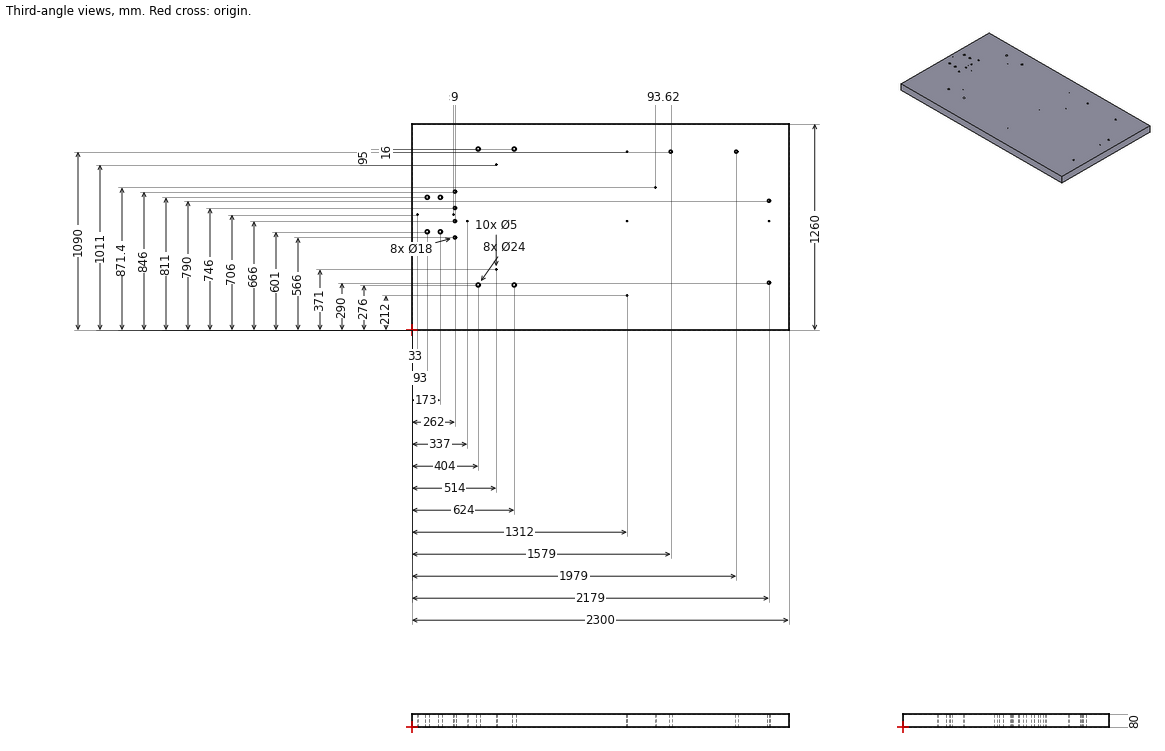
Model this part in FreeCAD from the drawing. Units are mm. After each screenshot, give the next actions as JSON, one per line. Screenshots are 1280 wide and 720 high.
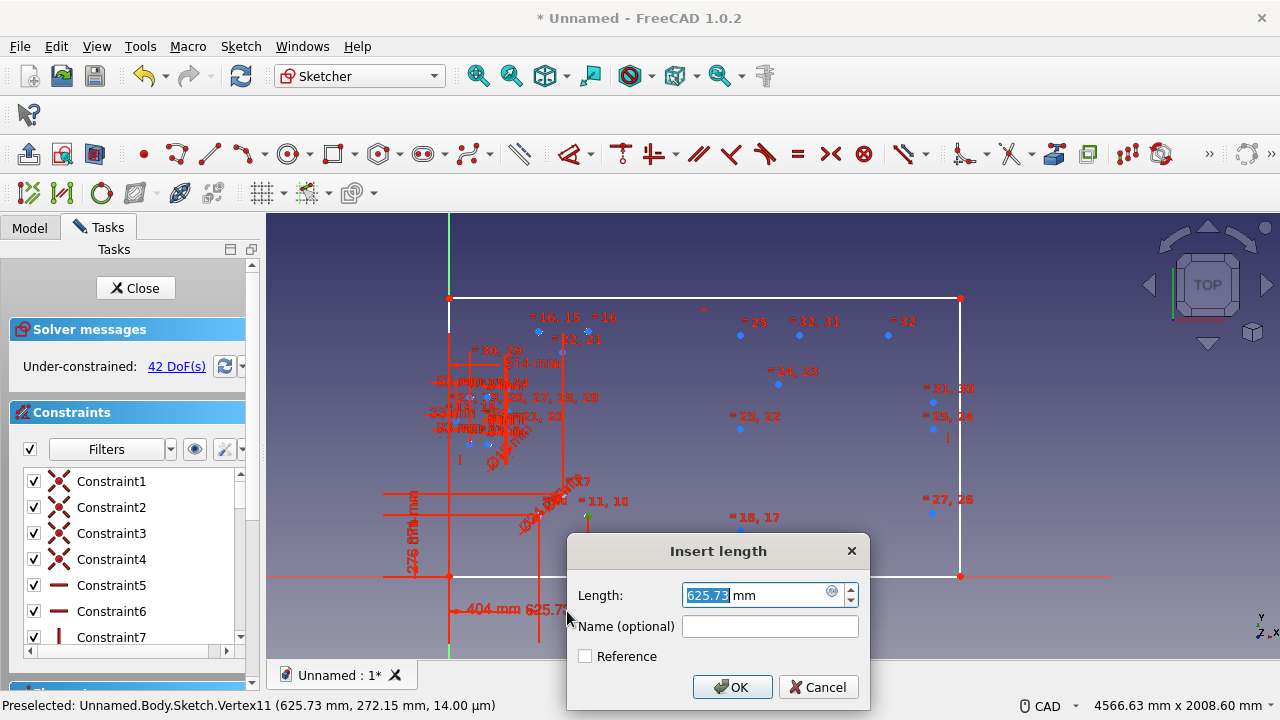
{"action": "type", "text": "624"}
{"action": "key", "text": "Return"}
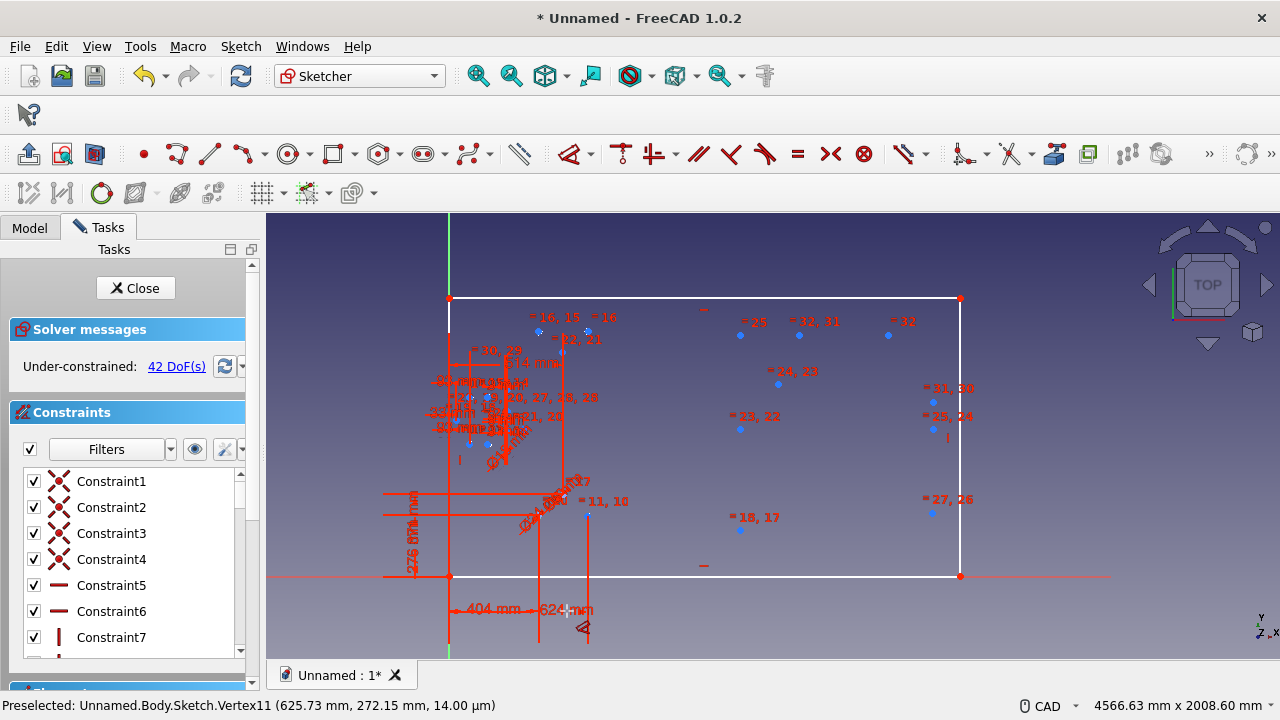
{"action": "left_click", "coordinate": [588, 516]}
{"action": "left_click", "coordinate": [622, 546]}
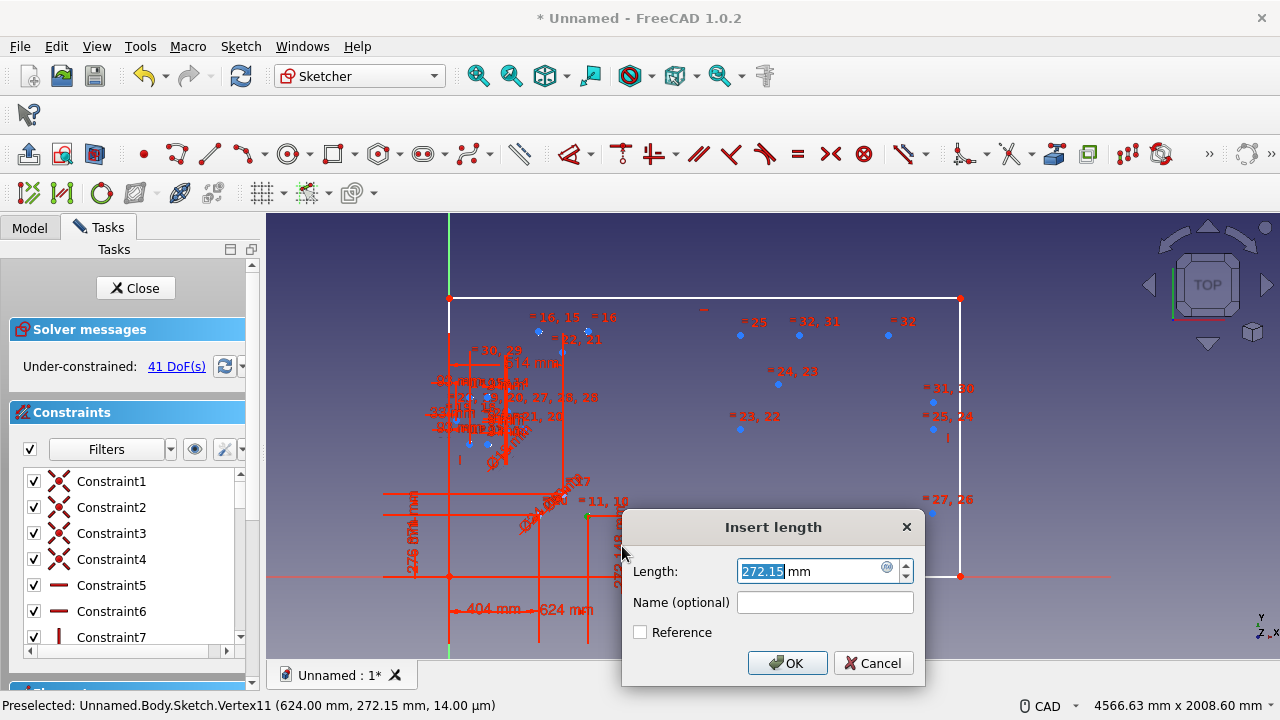
{"action": "type", "text": "276"}
{"action": "key", "text": "Return"}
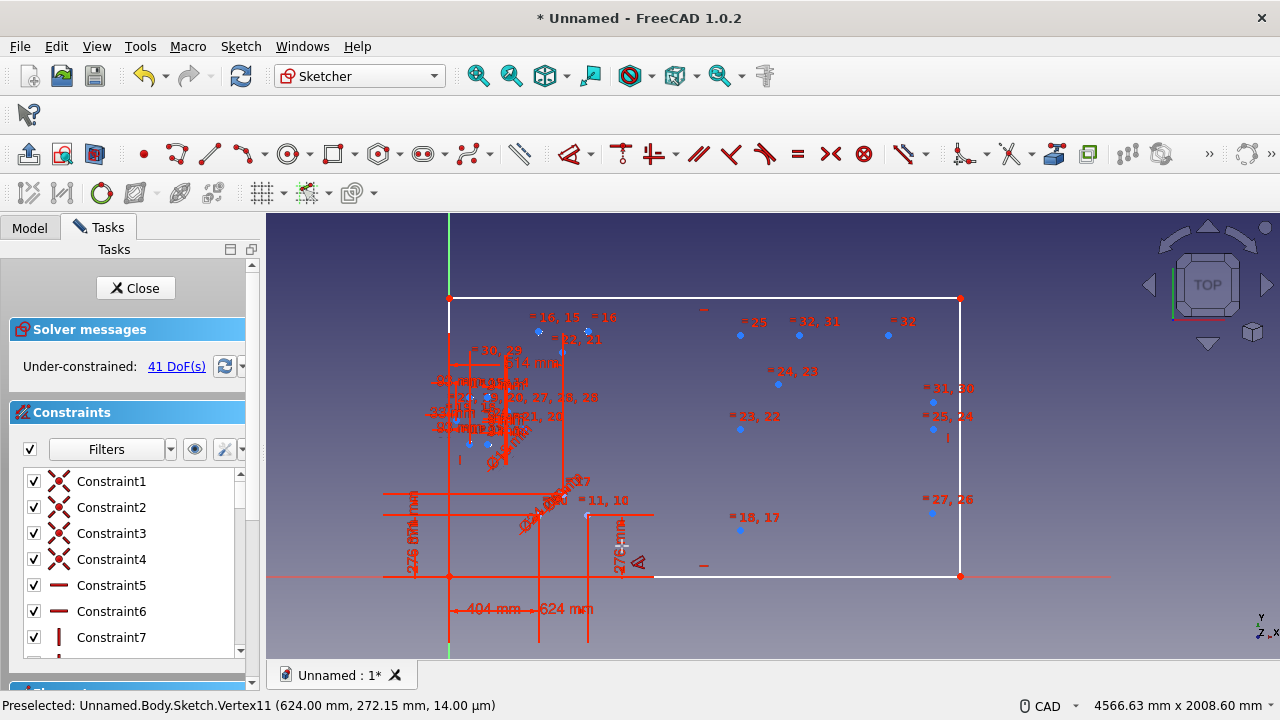
{"action": "left_click", "coordinate": [470, 444]}
{"action": "left_click", "coordinate": [415, 480]}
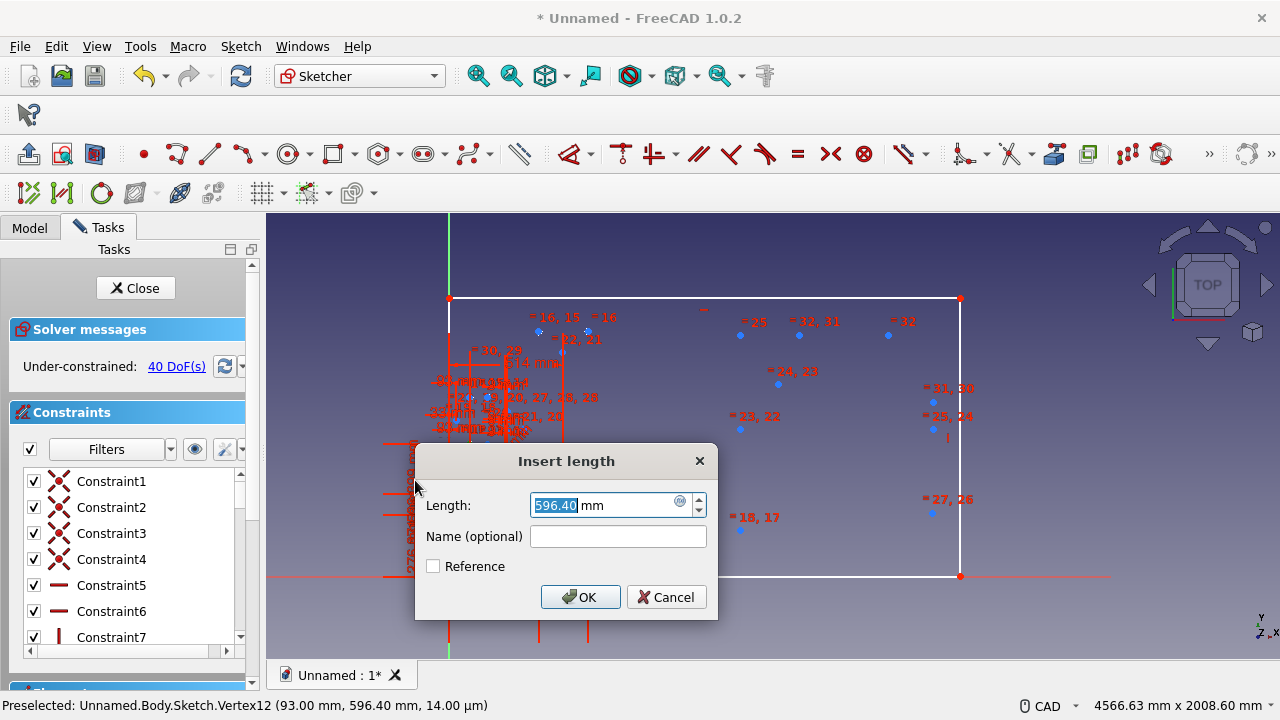
{"action": "type", "text": "601"}
{"action": "key", "text": "Return"}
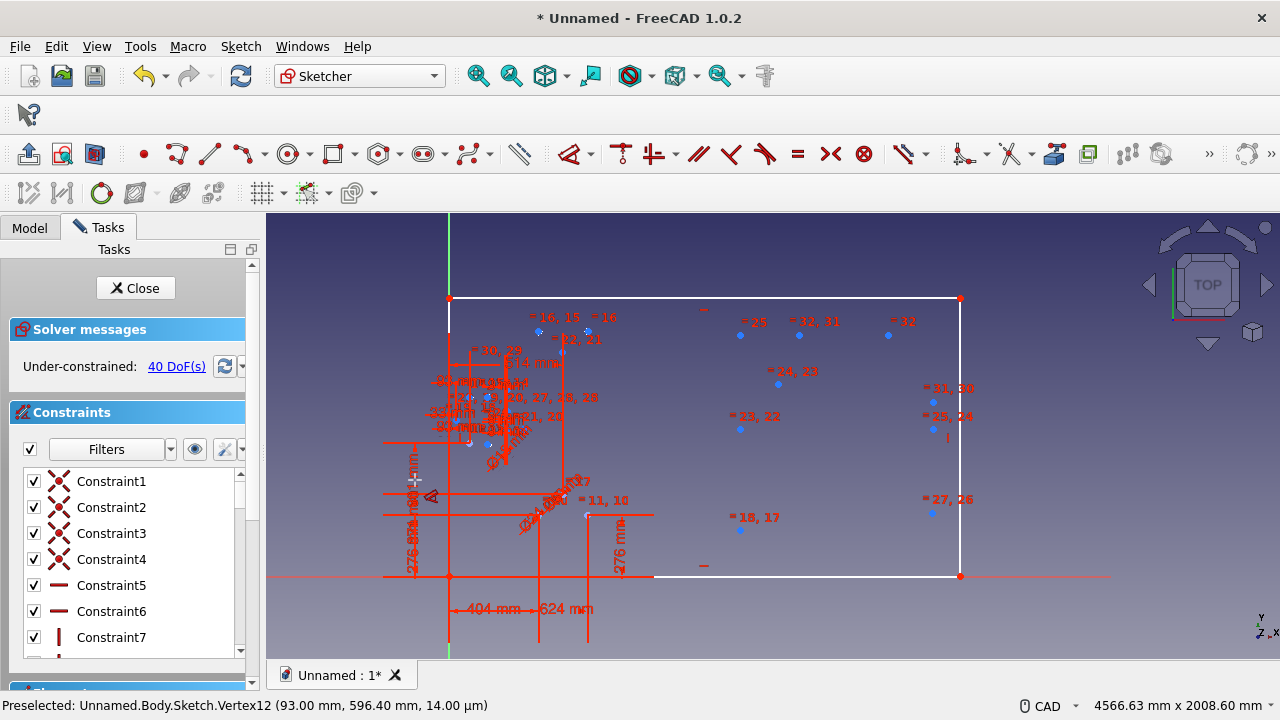
{"action": "left_click", "coordinate": [507, 452]}
{"action": "left_click", "coordinate": [478, 322]}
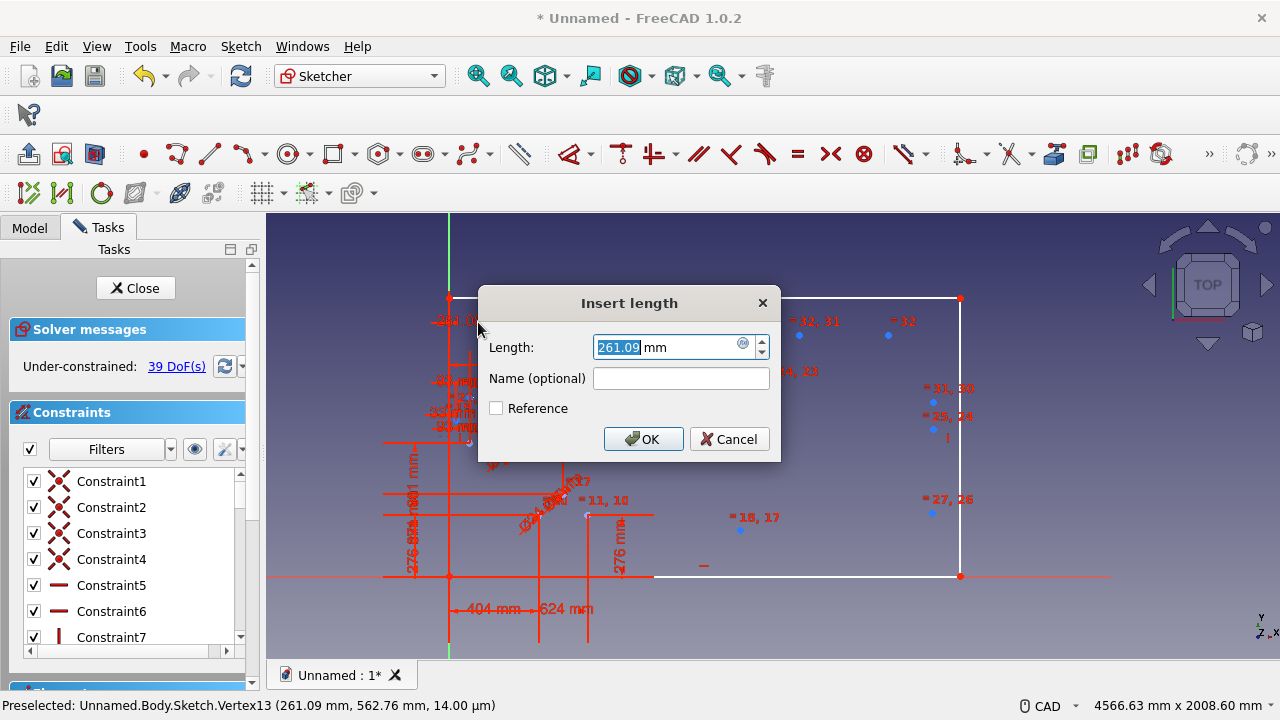
{"action": "type", "text": "262"}
{"action": "key", "text": "Return"}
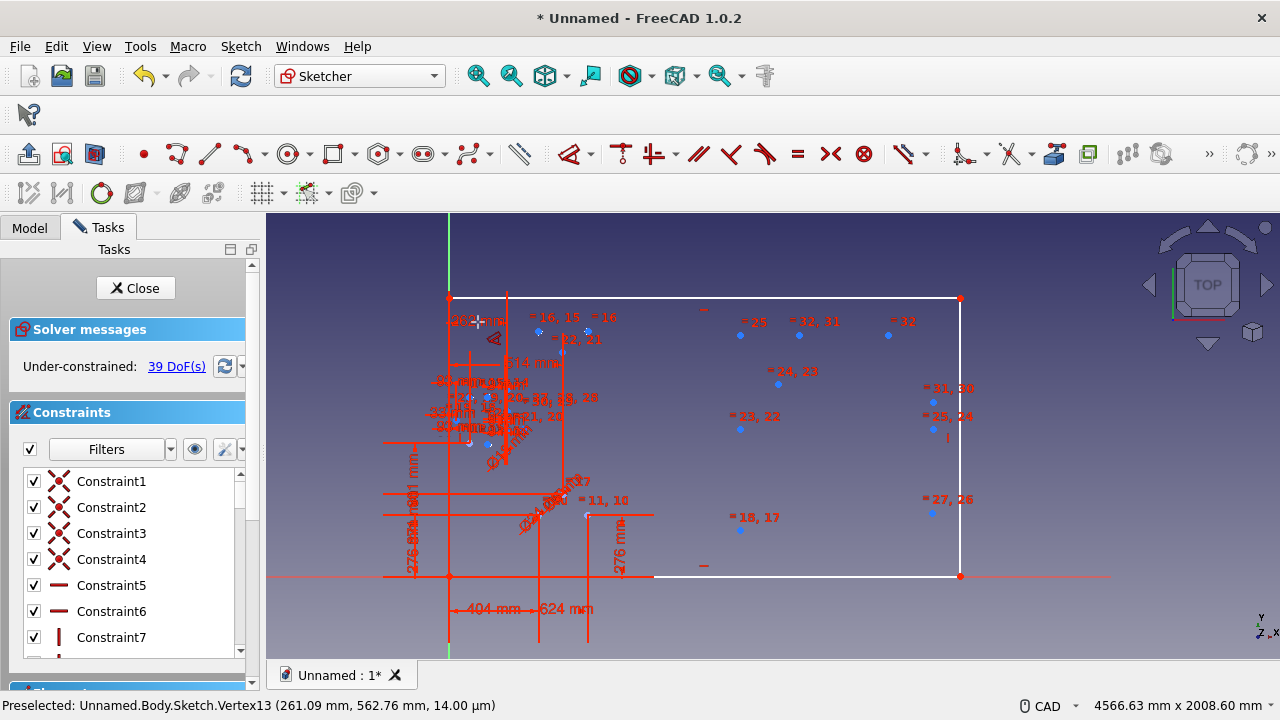
{"action": "left_click", "coordinate": [507, 452]}
{"action": "left_click", "coordinate": [541, 543]}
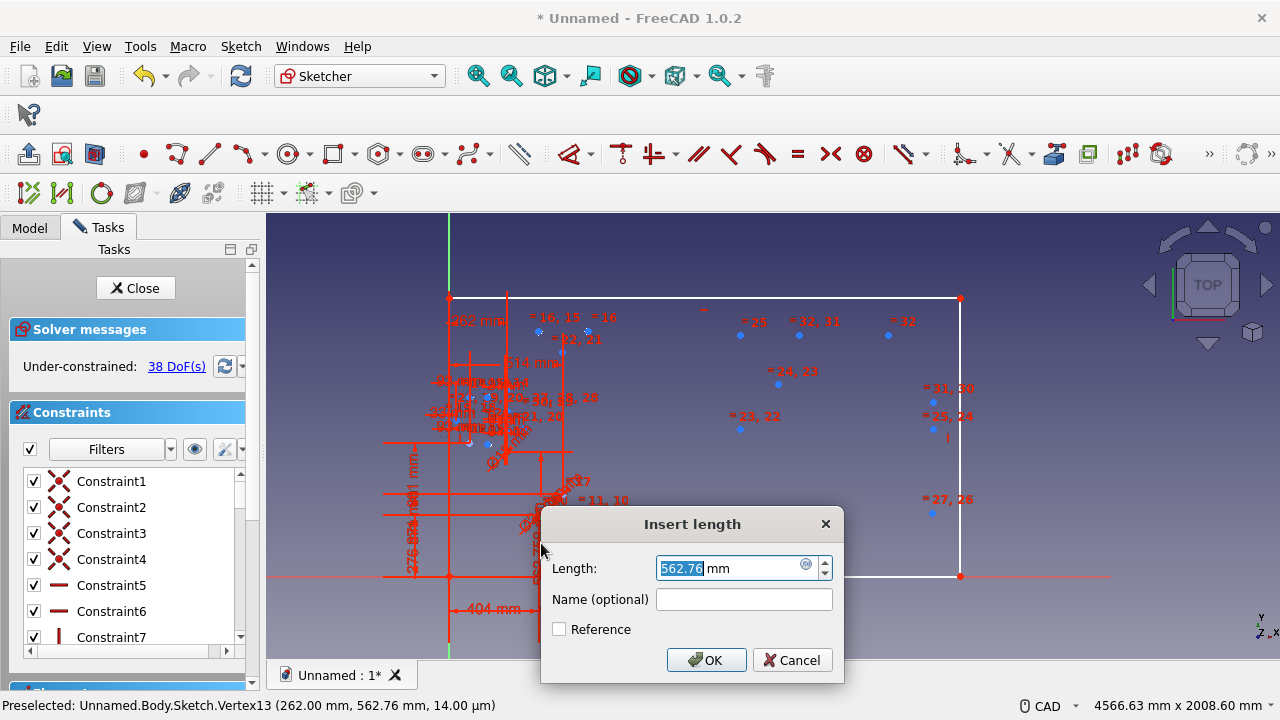
{"action": "type", "text": "566"}
{"action": "key", "text": "Return"}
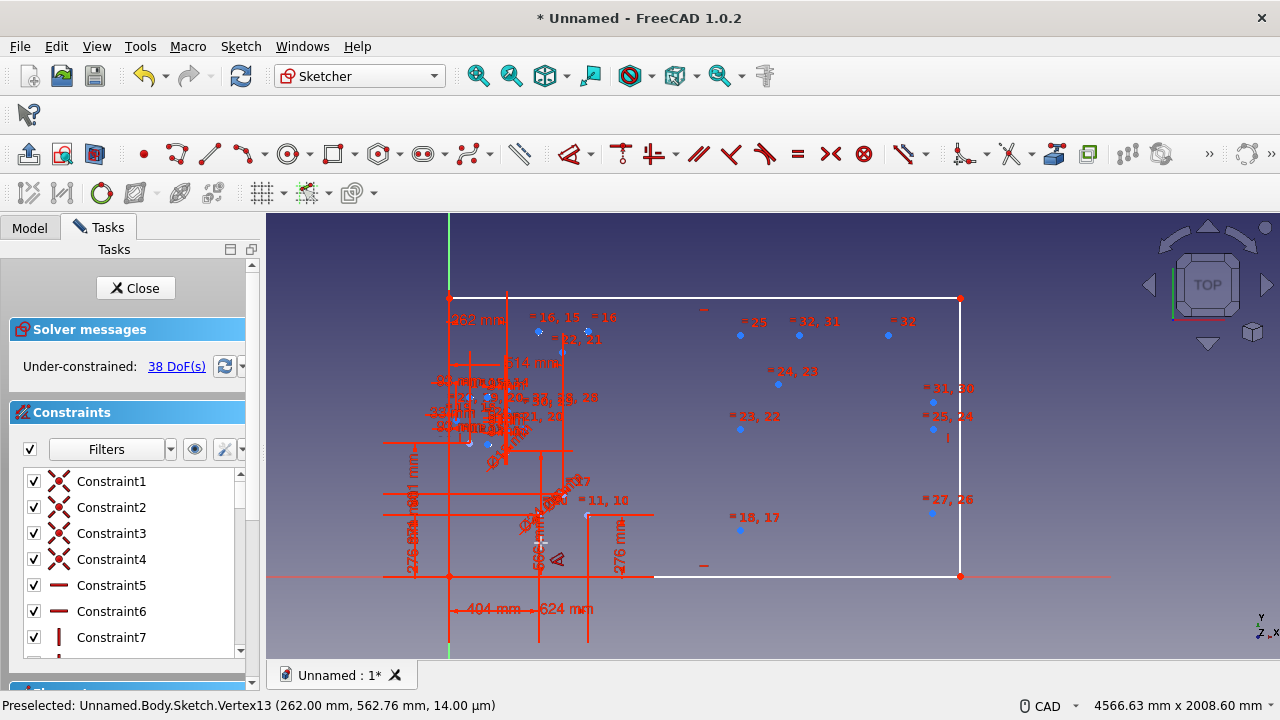
{"action": "left_click", "coordinate": [488, 445]}
{"action": "left_click", "coordinate": [469, 265]}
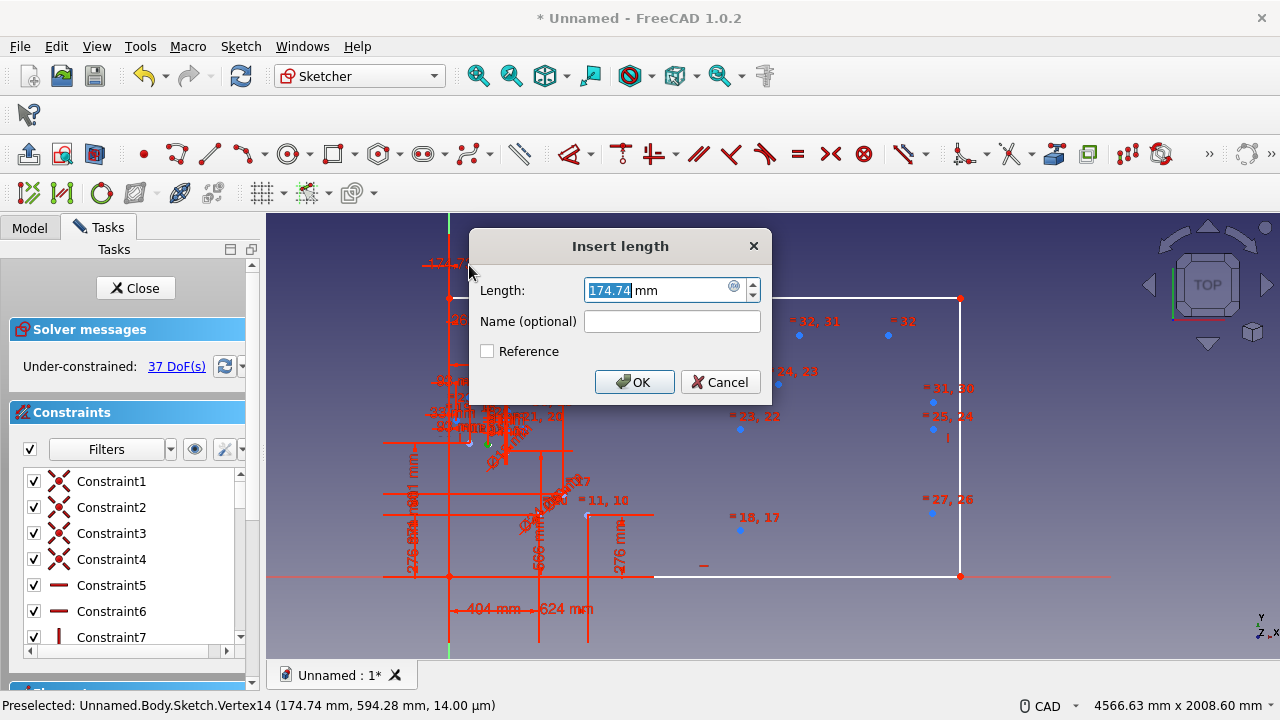
{"action": "type", "text": "173"}
{"action": "key", "text": "Return"}